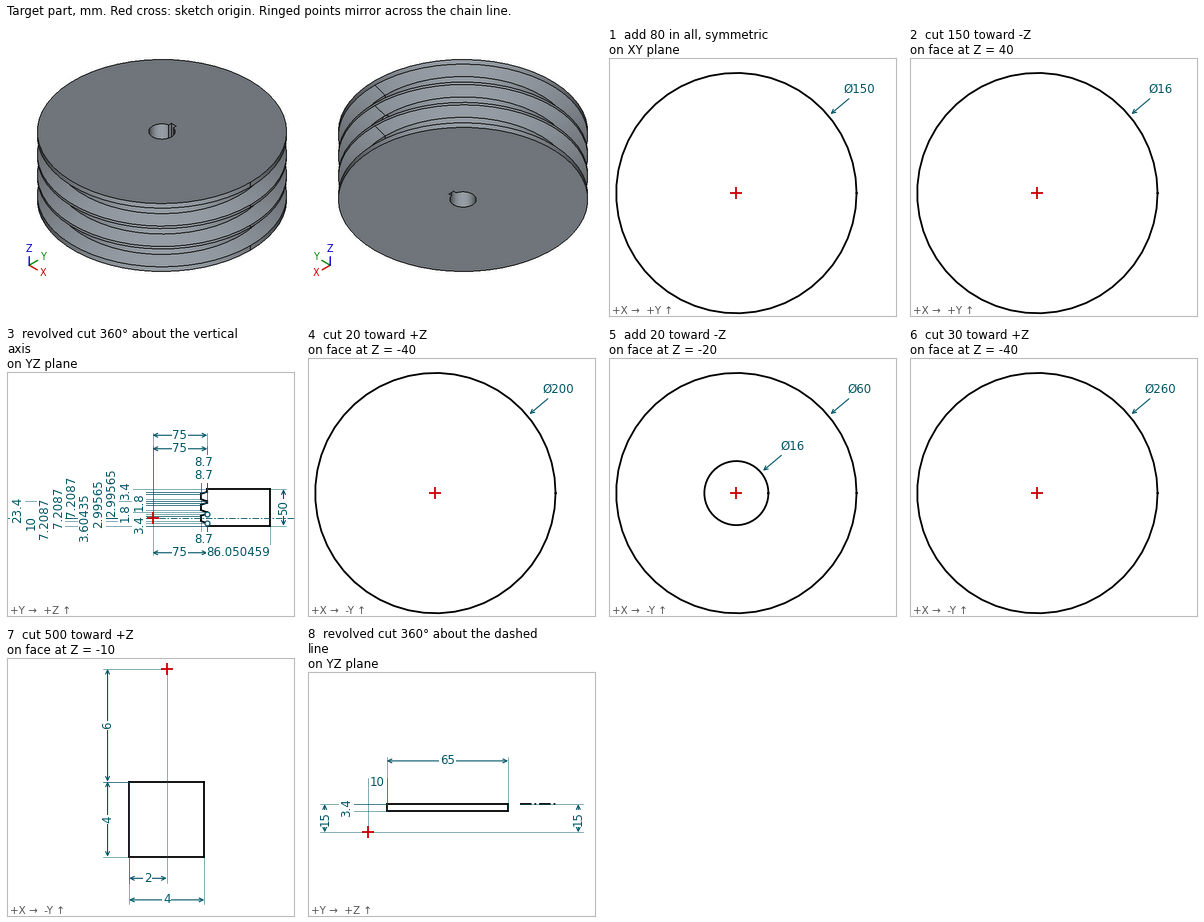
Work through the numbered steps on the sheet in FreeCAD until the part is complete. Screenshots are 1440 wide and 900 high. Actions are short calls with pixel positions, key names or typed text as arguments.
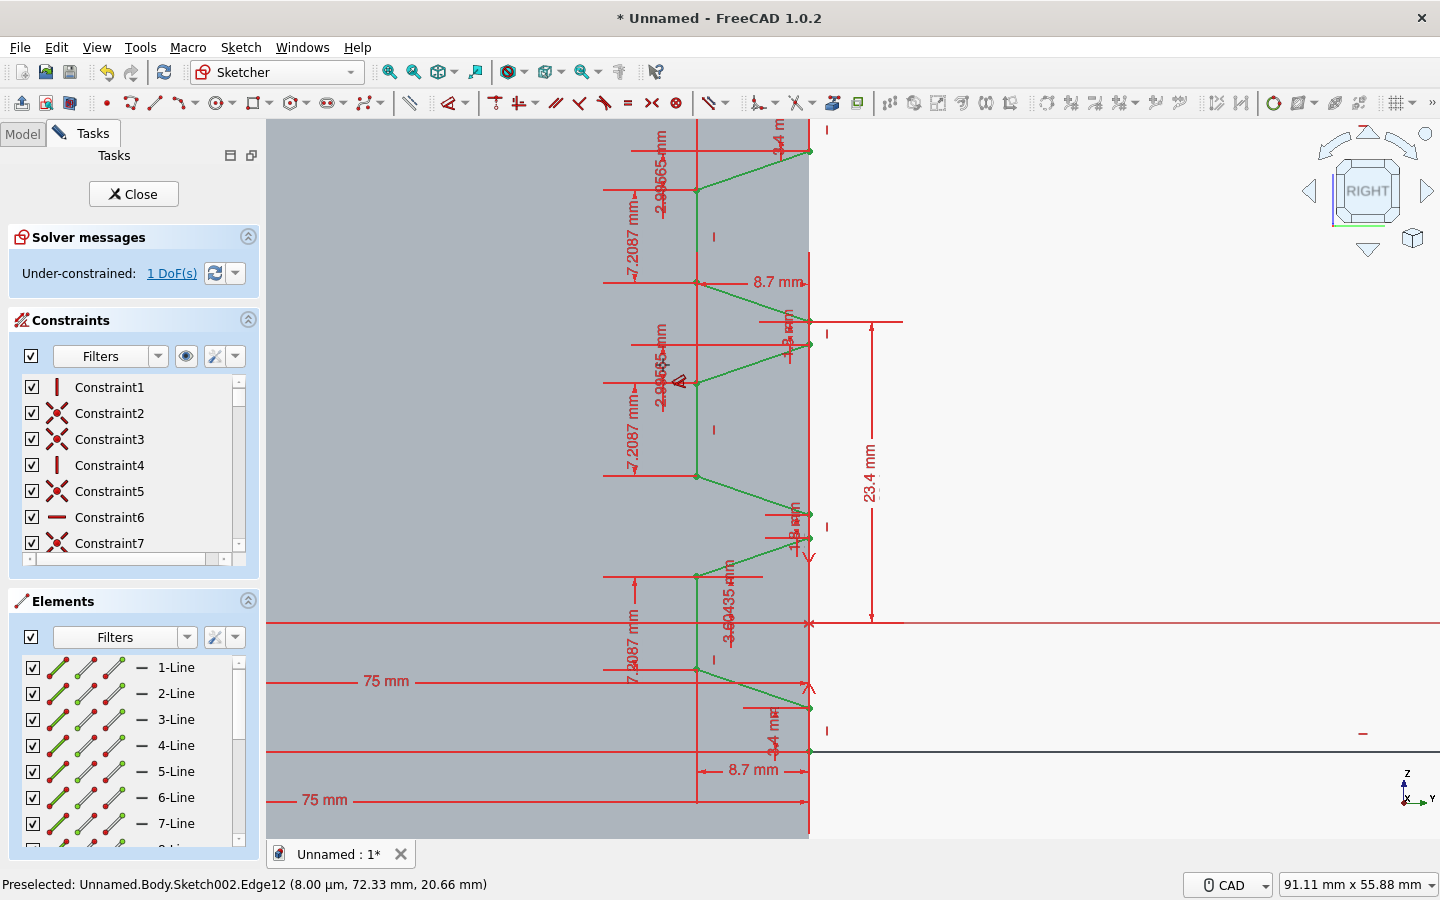
click(1142, 752)
click(1042, 786)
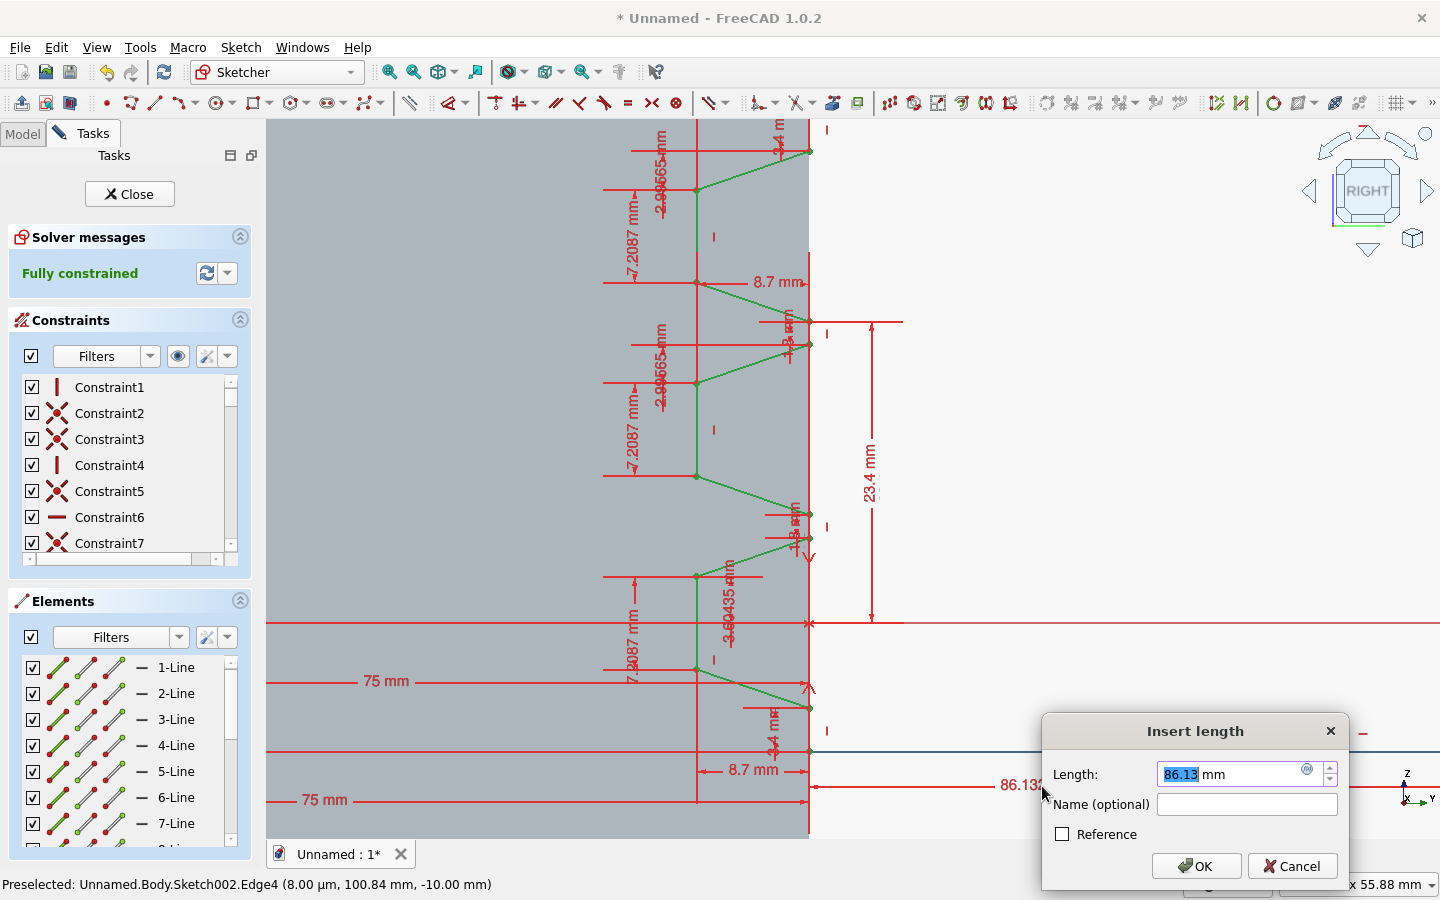
text(86.050459)
key(Return)
key(Escape)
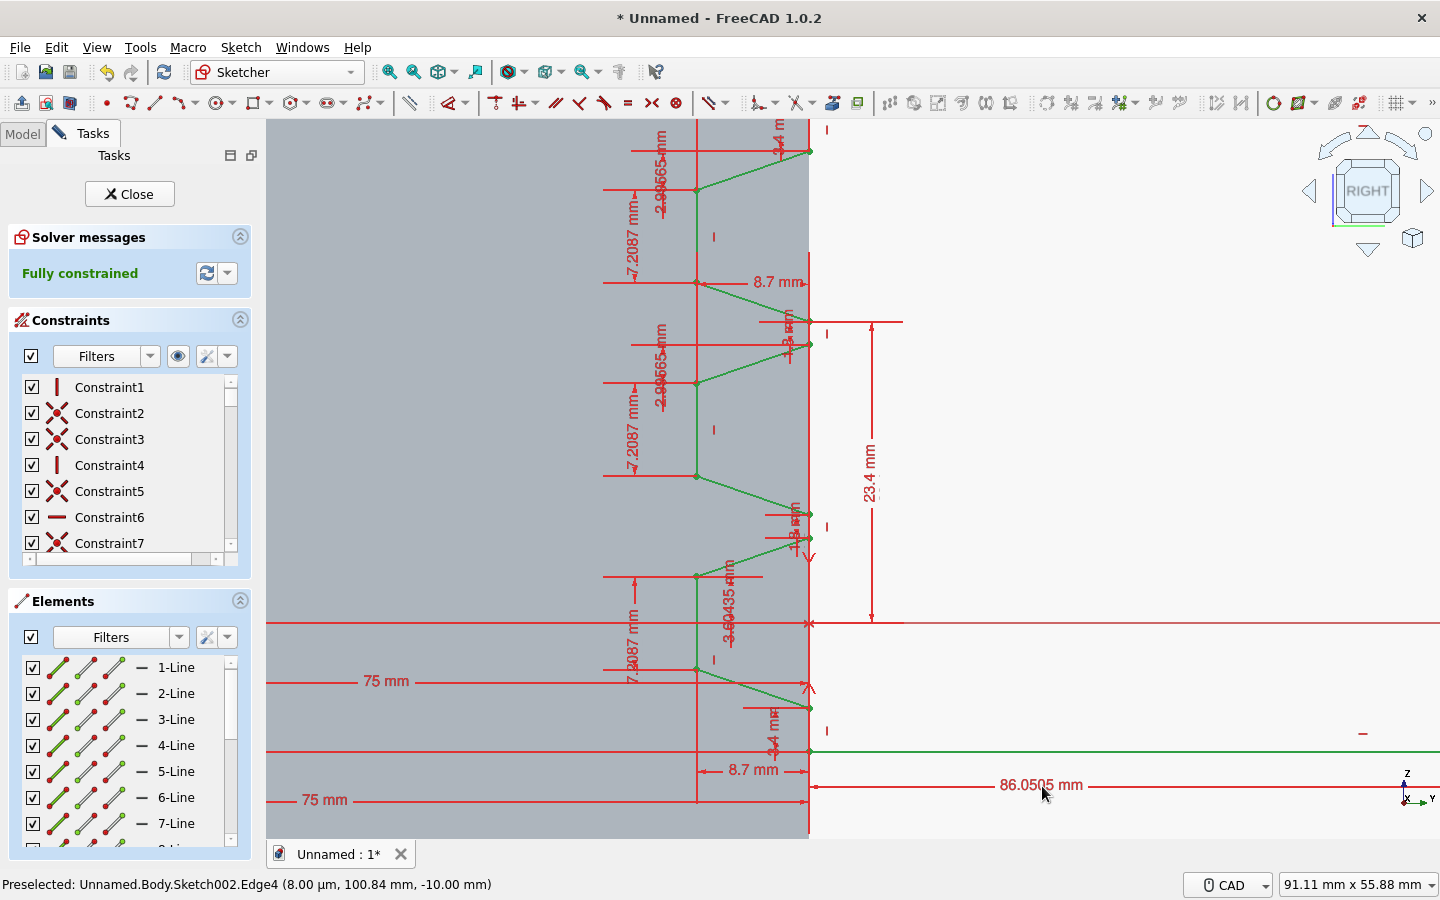
click(130, 194)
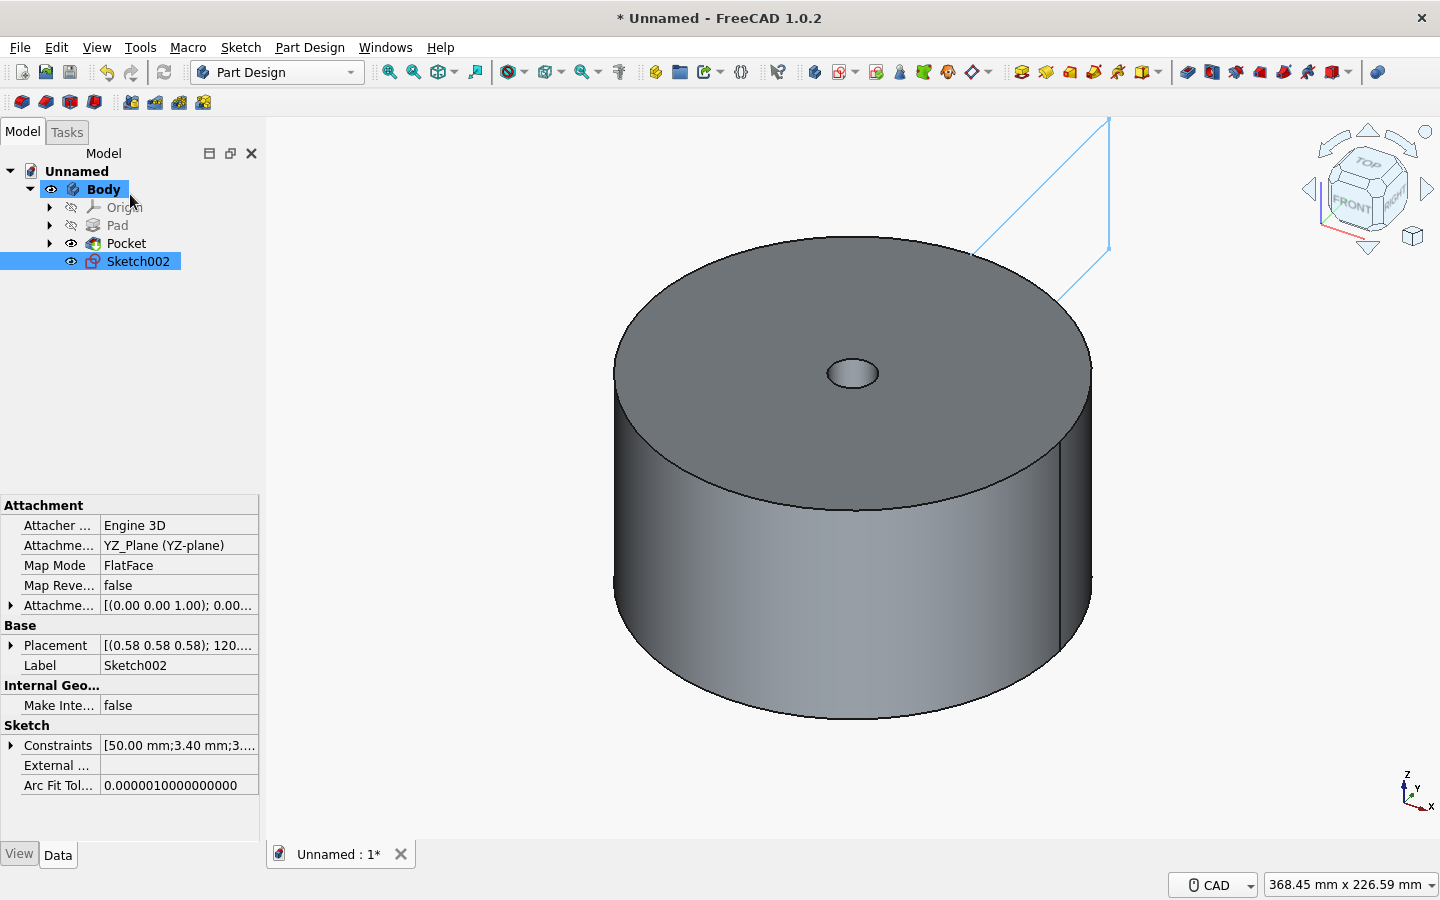
click(1236, 72)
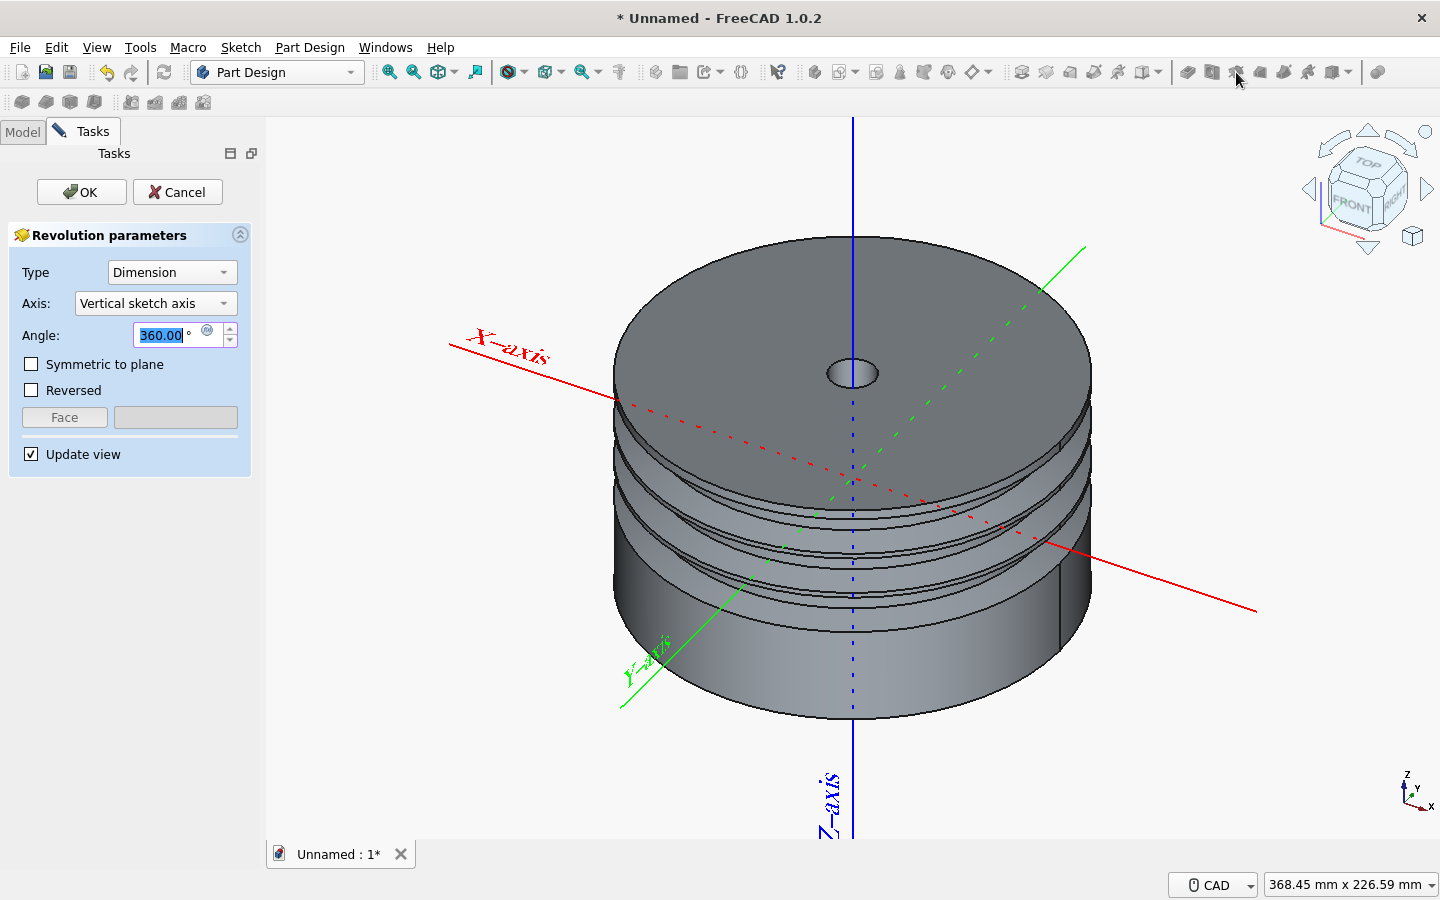
click(82, 192)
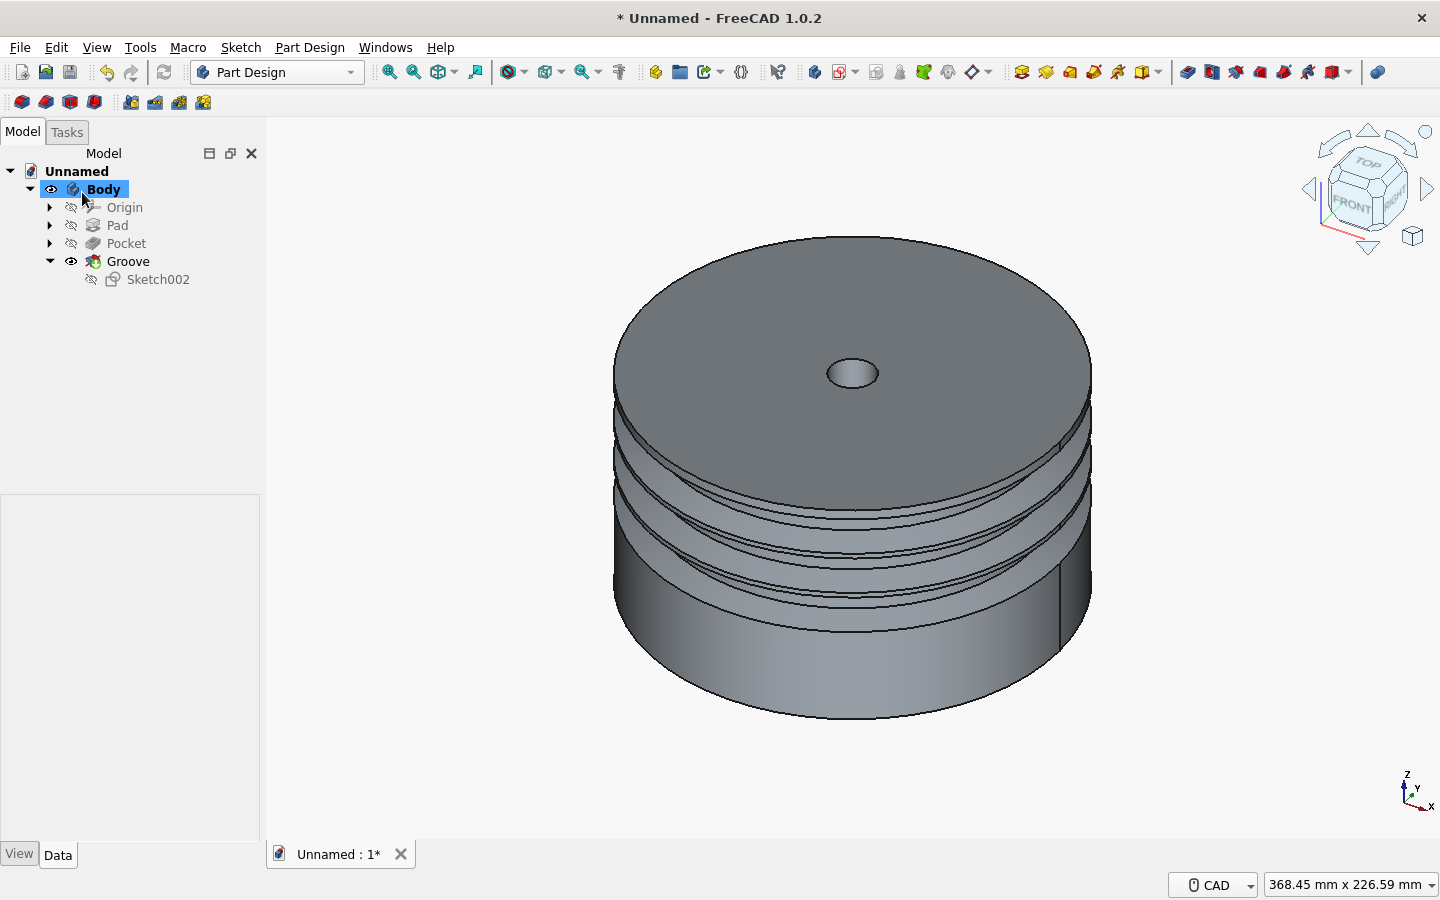
key(5)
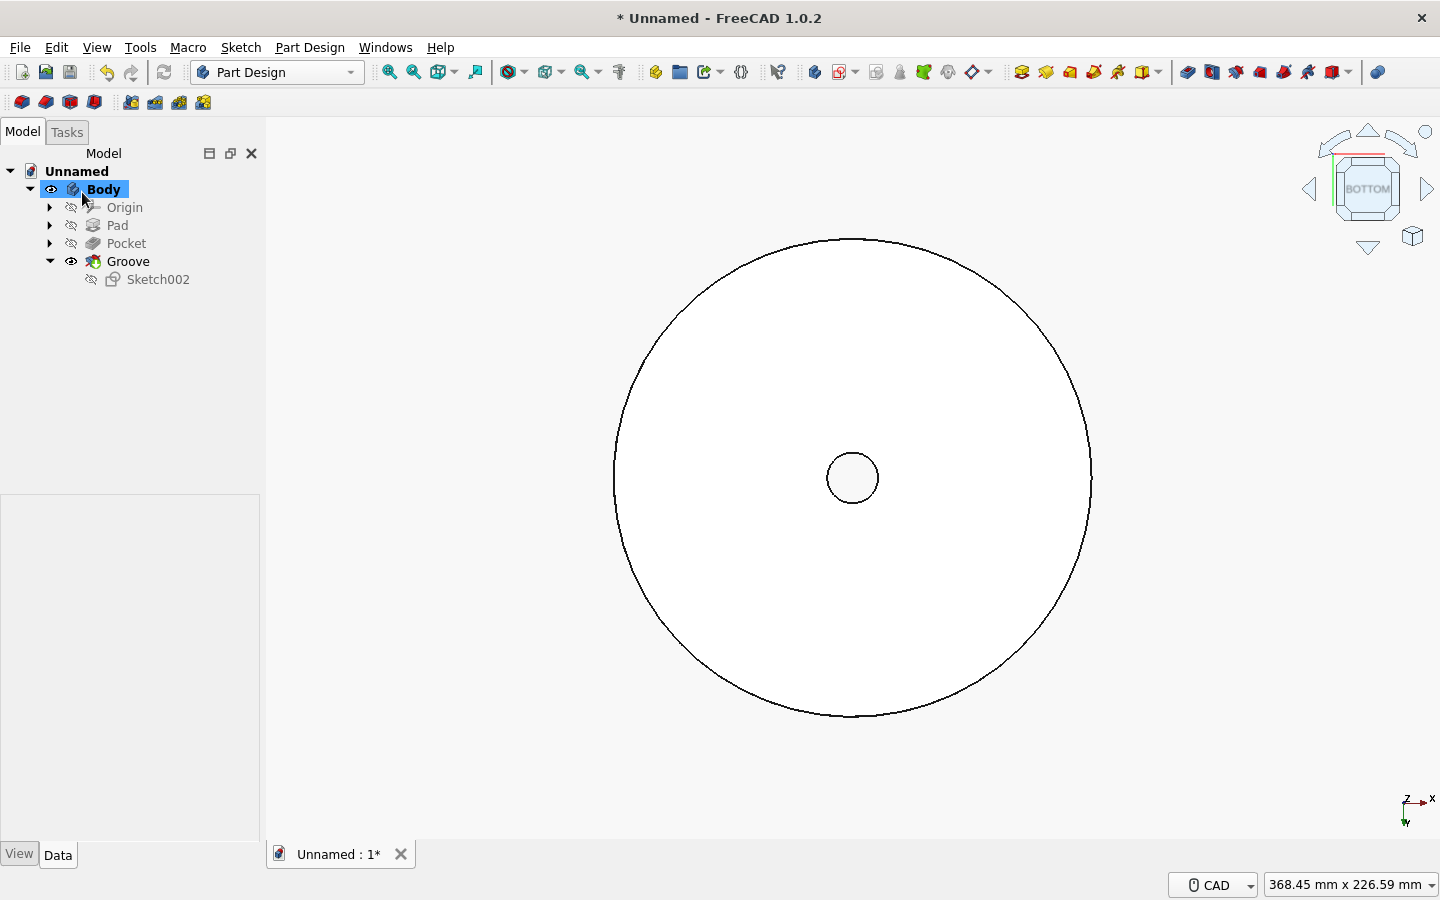
click(989, 477)